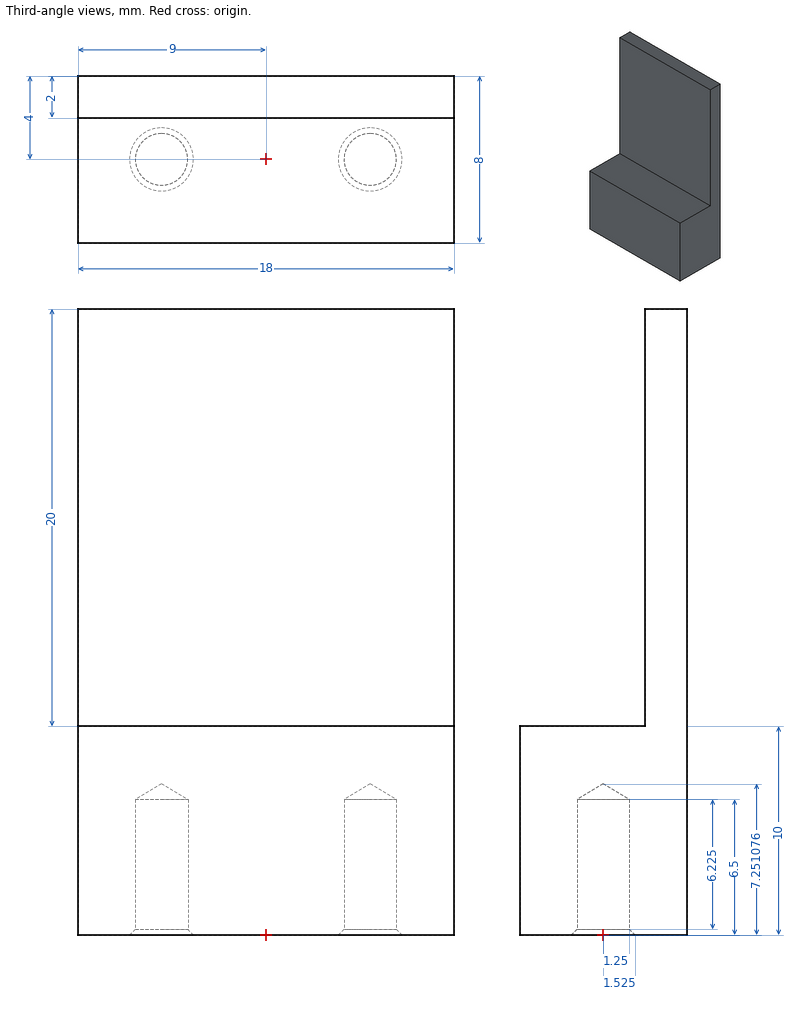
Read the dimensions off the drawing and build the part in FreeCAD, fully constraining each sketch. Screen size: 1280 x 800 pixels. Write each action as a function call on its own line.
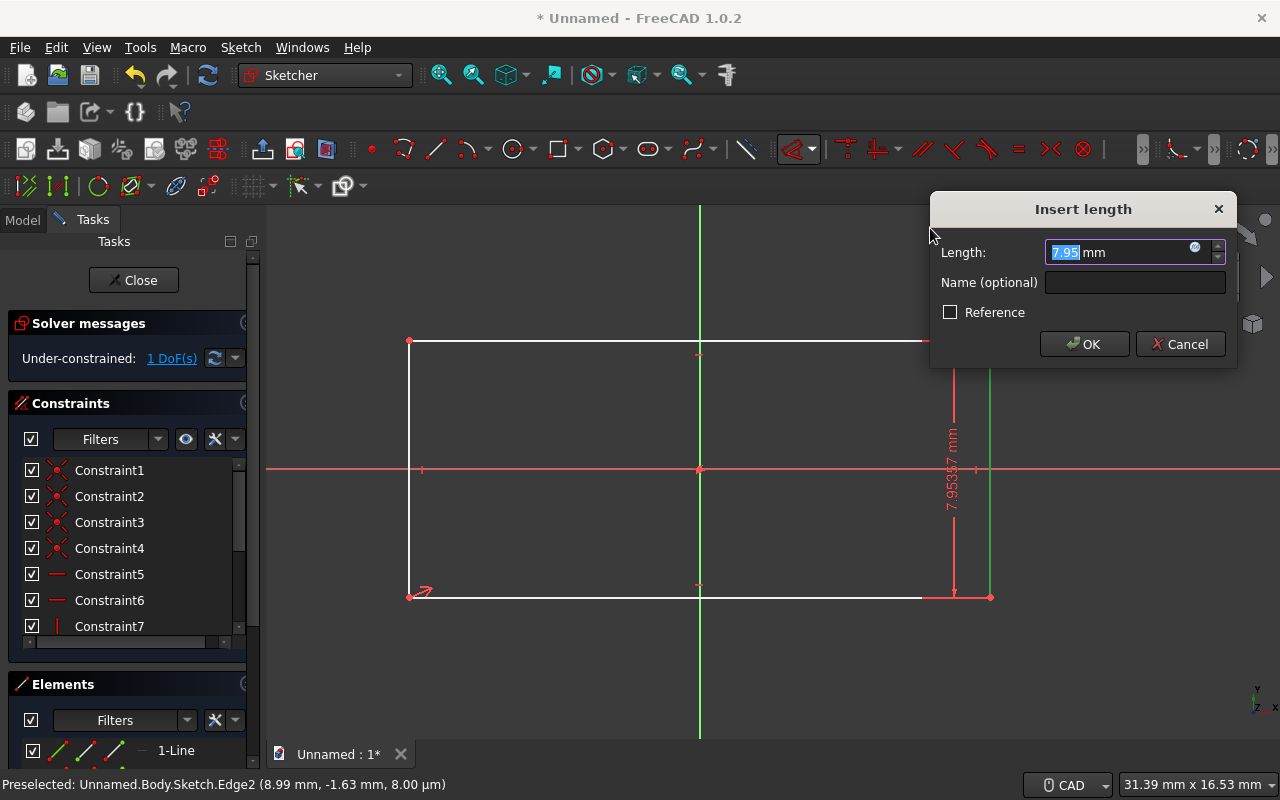
text(8)
key(Return)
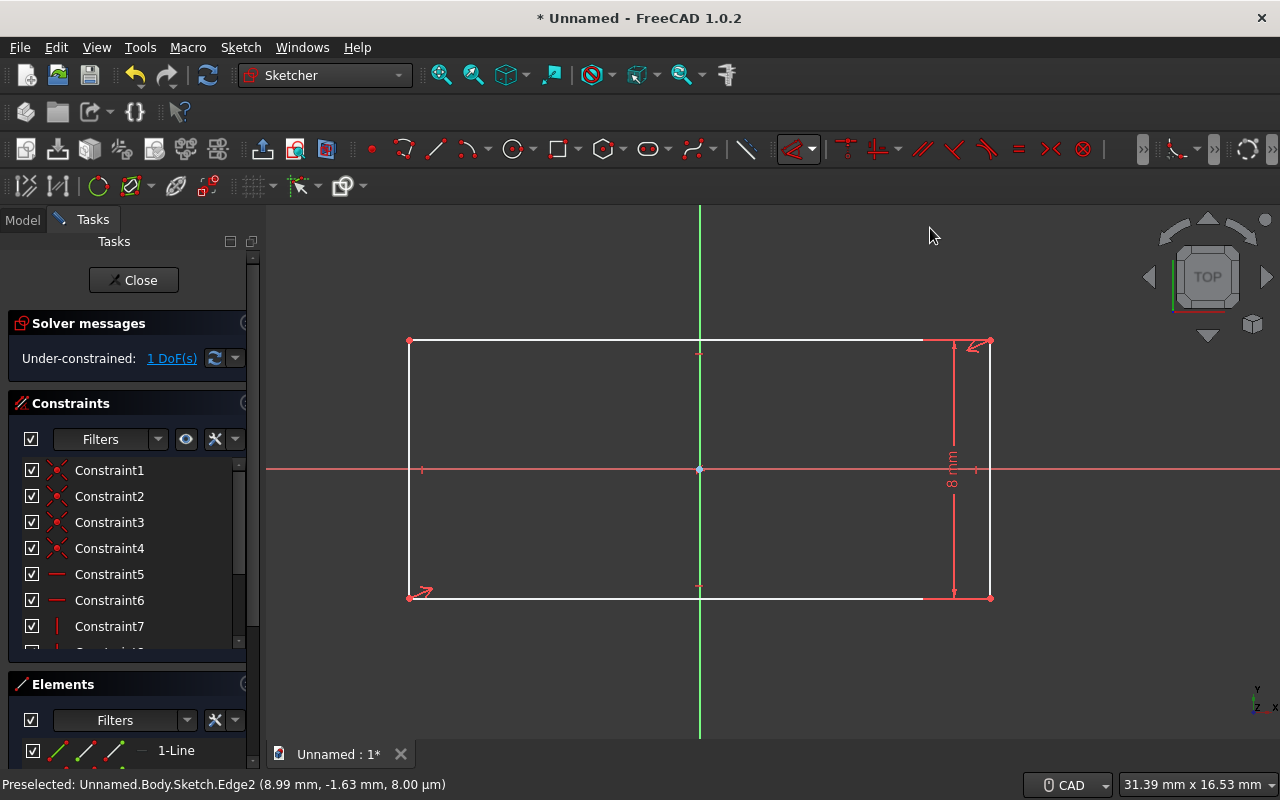
click(584, 599)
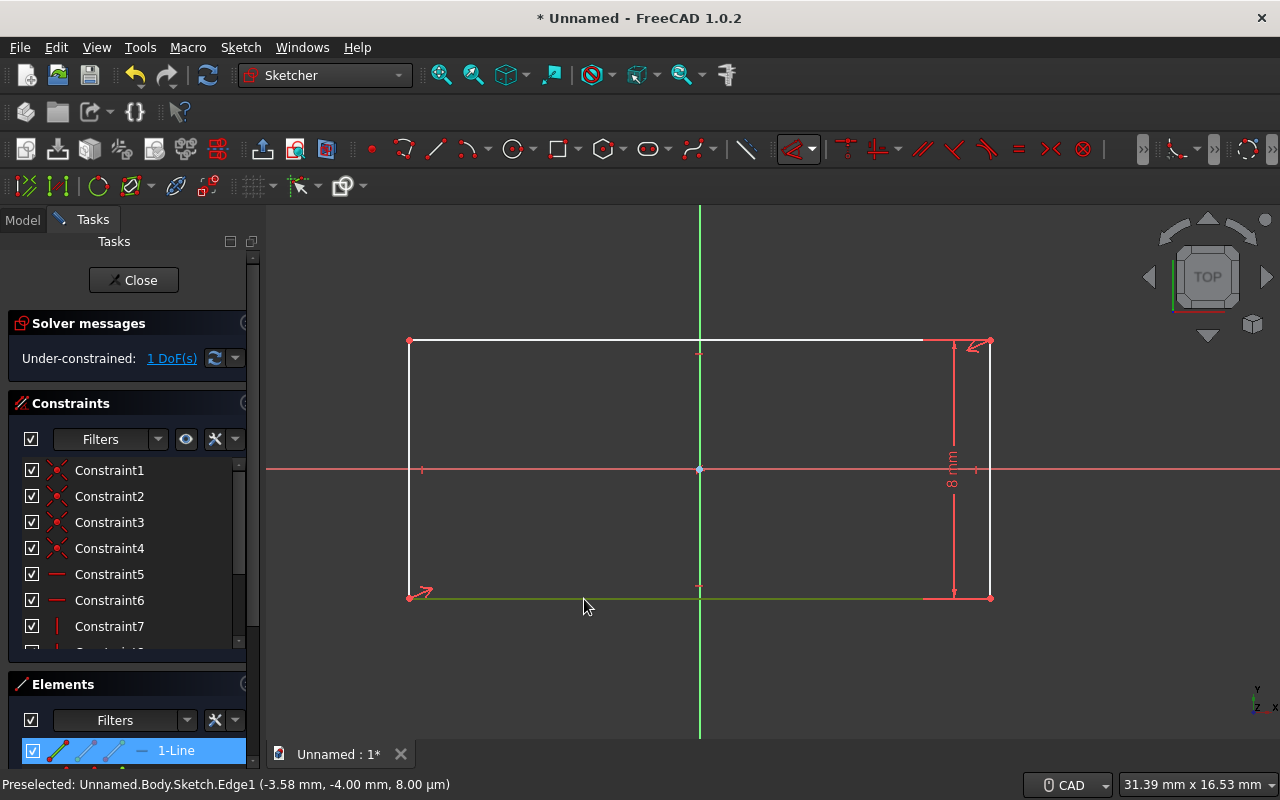
key(l)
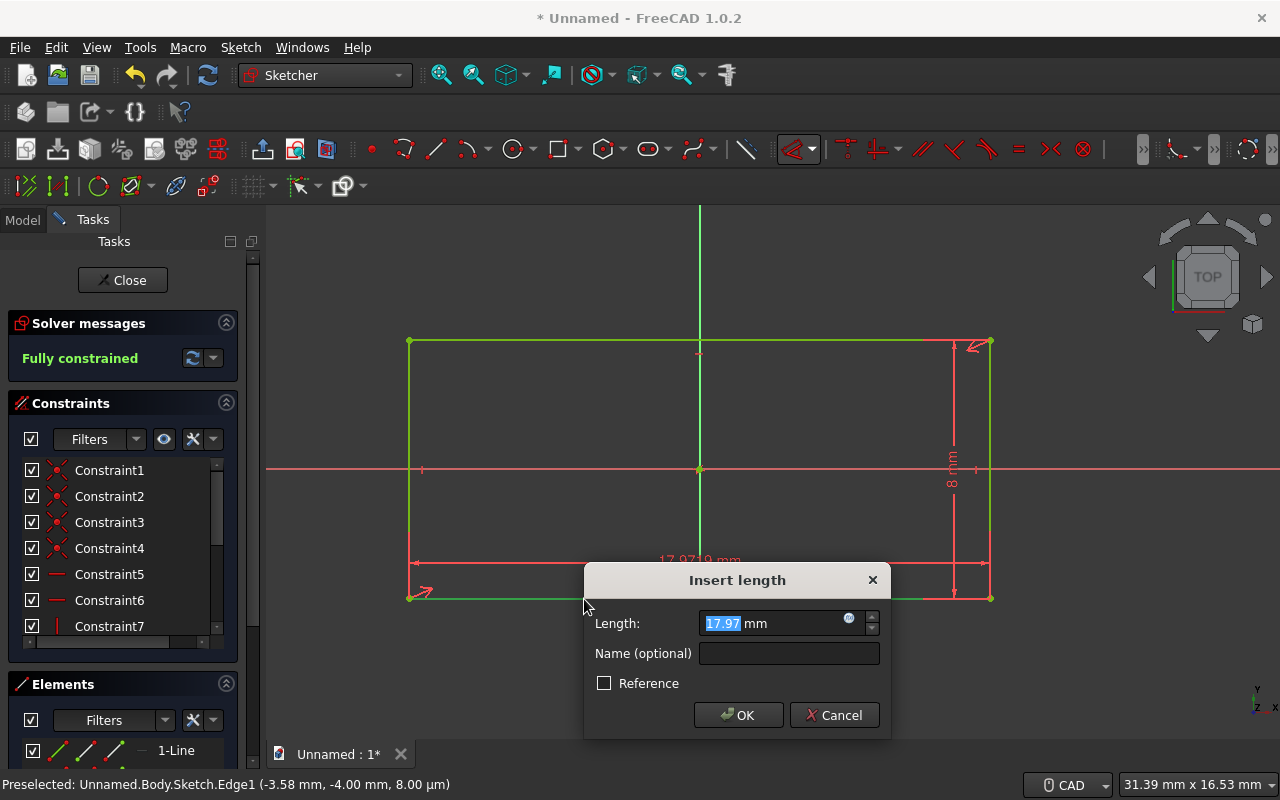
text(18)
key(Return)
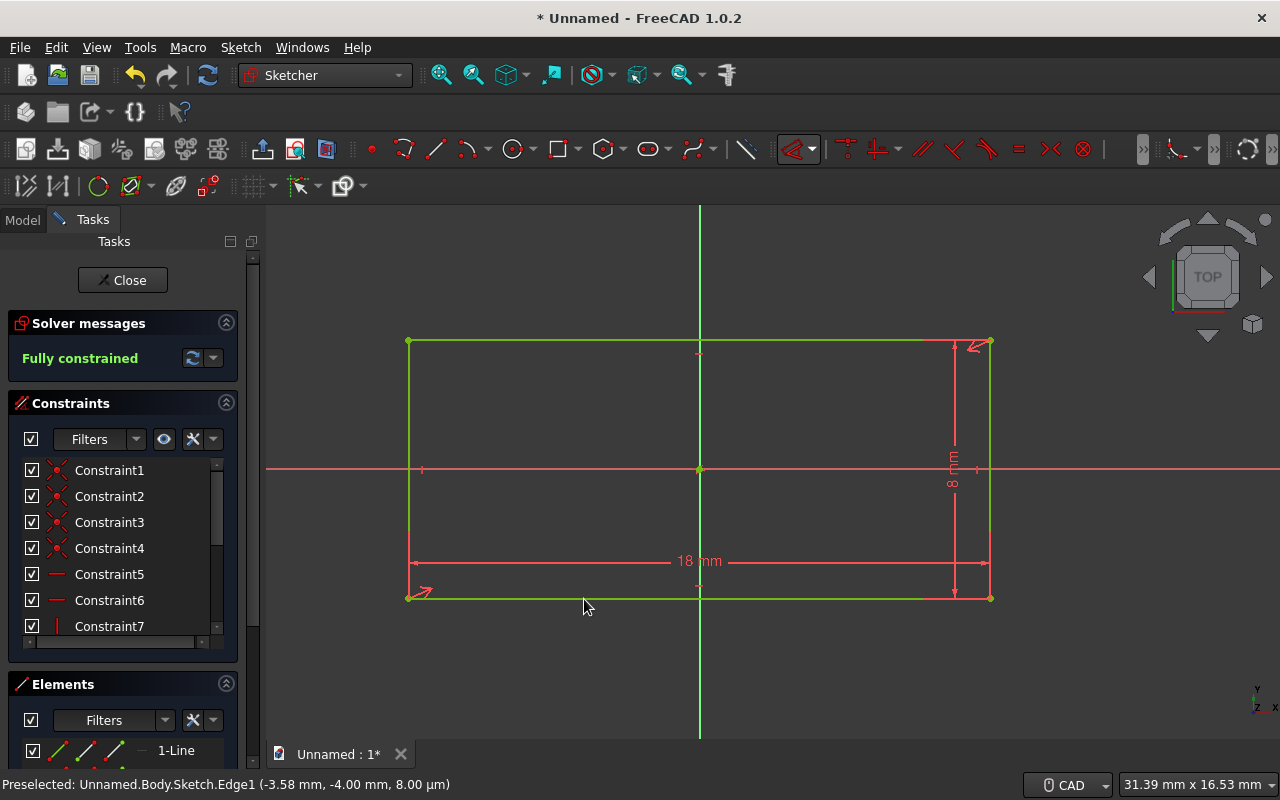
click(123, 280)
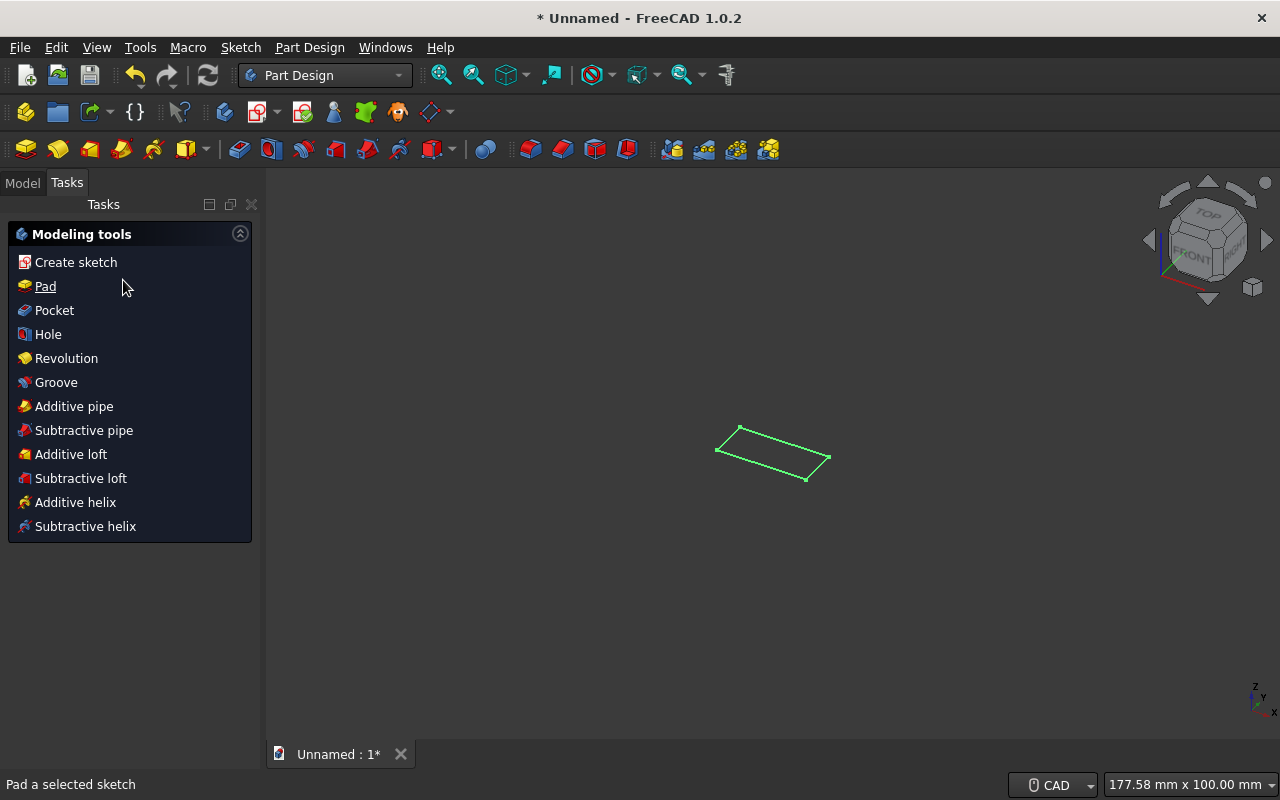
click(26, 150)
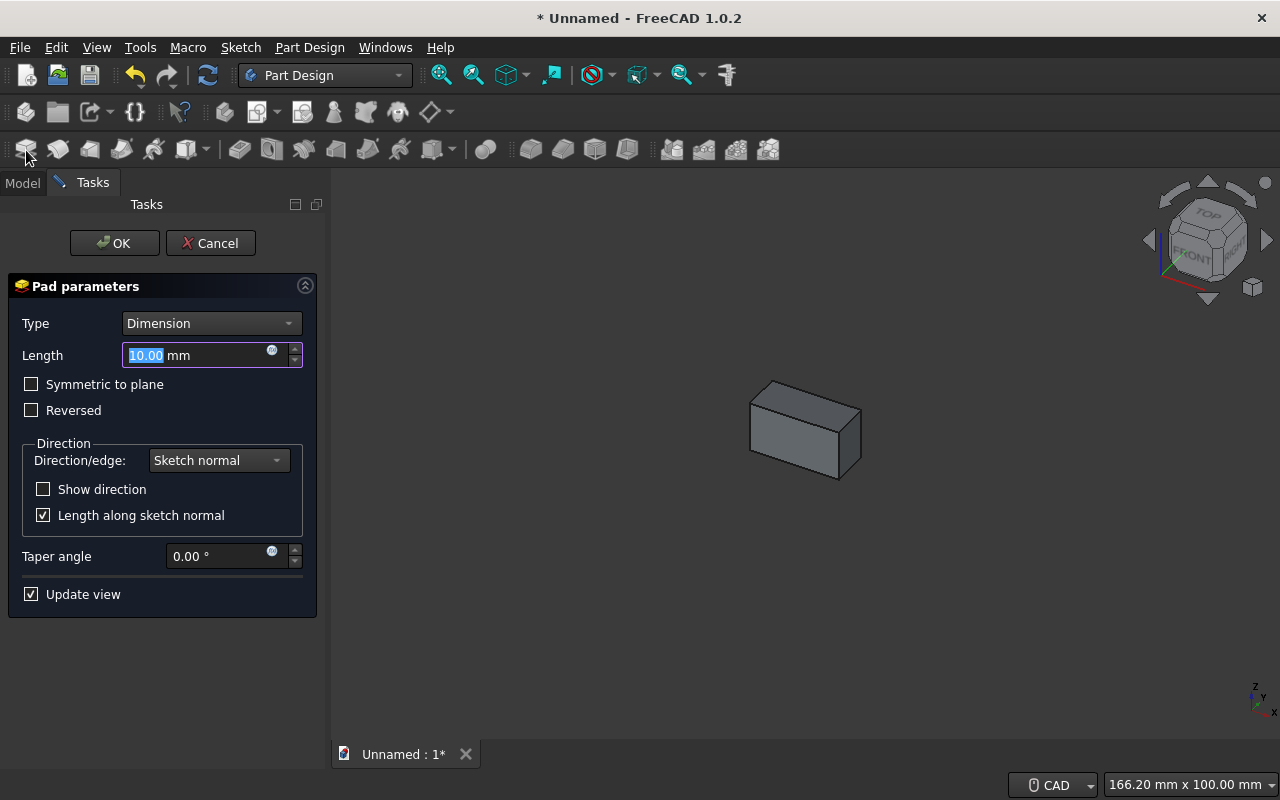
text(10)
key(Tab)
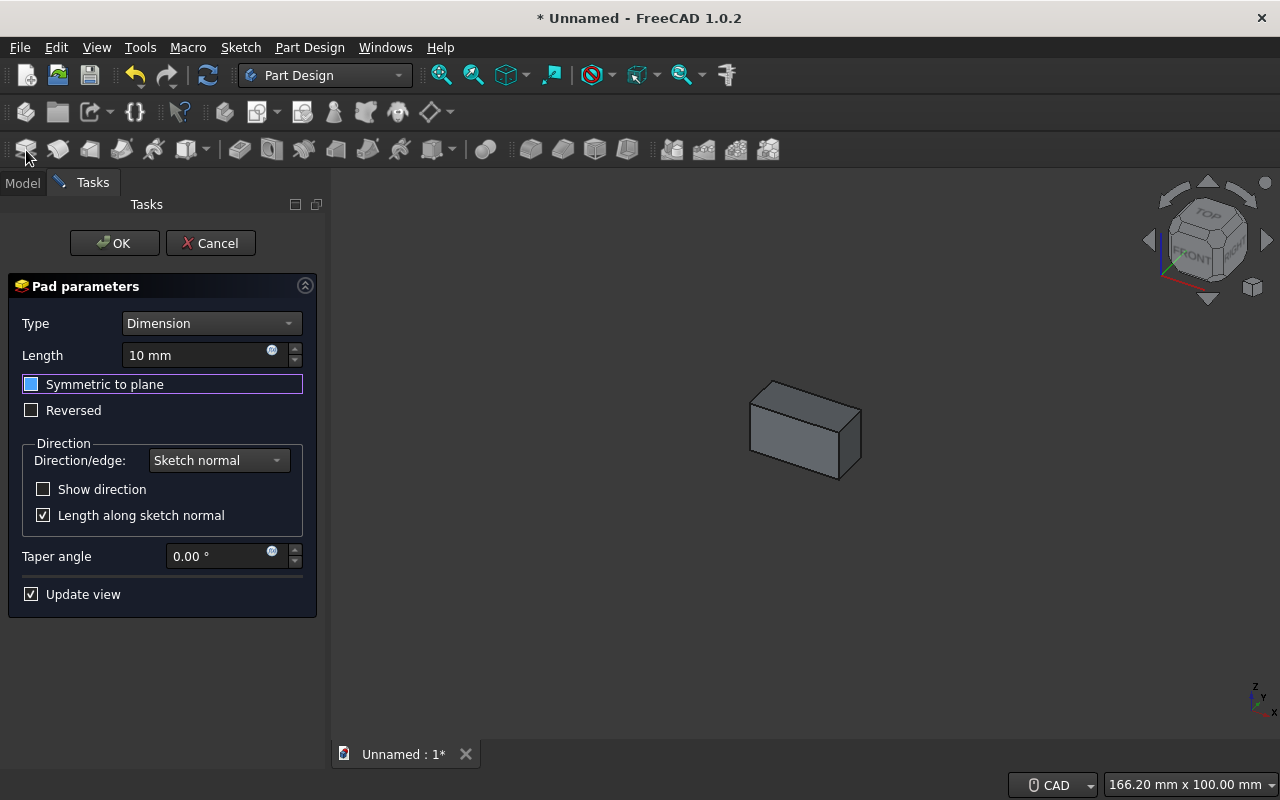
click(115, 243)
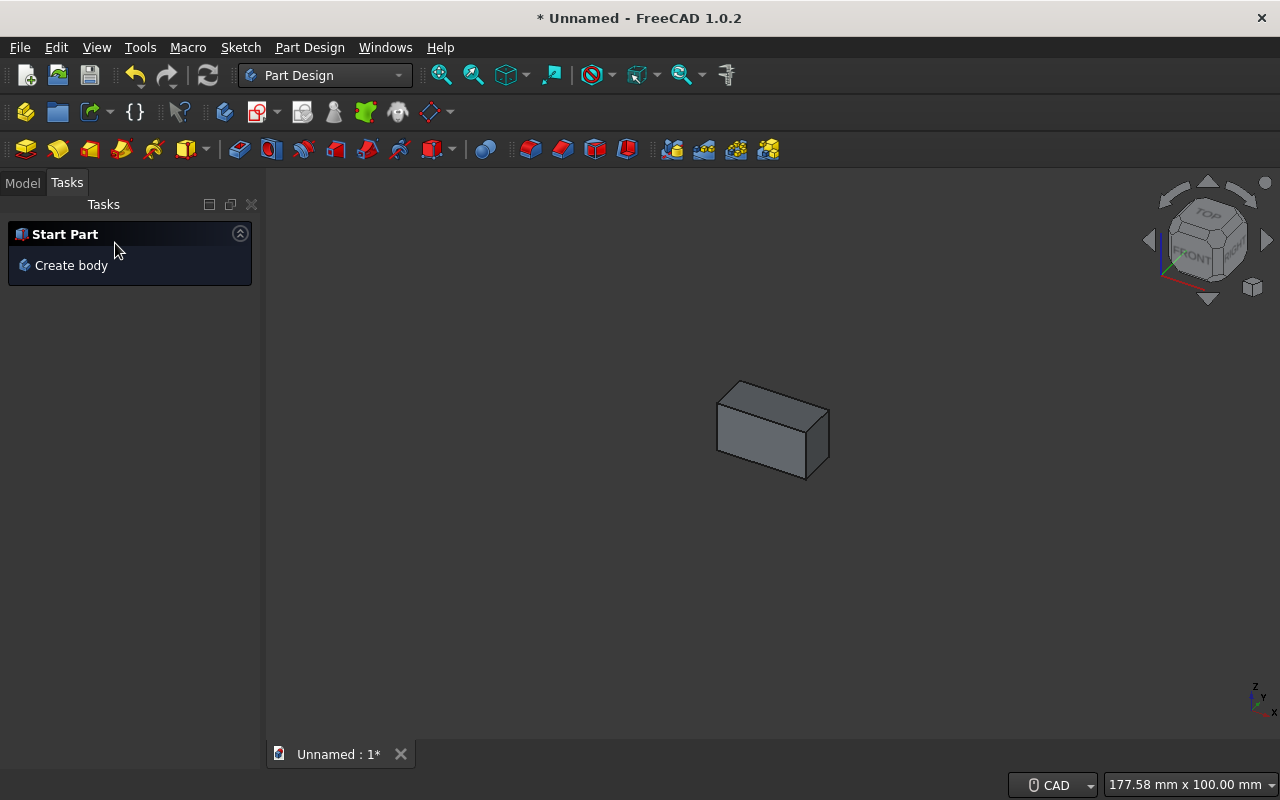
click(442, 76)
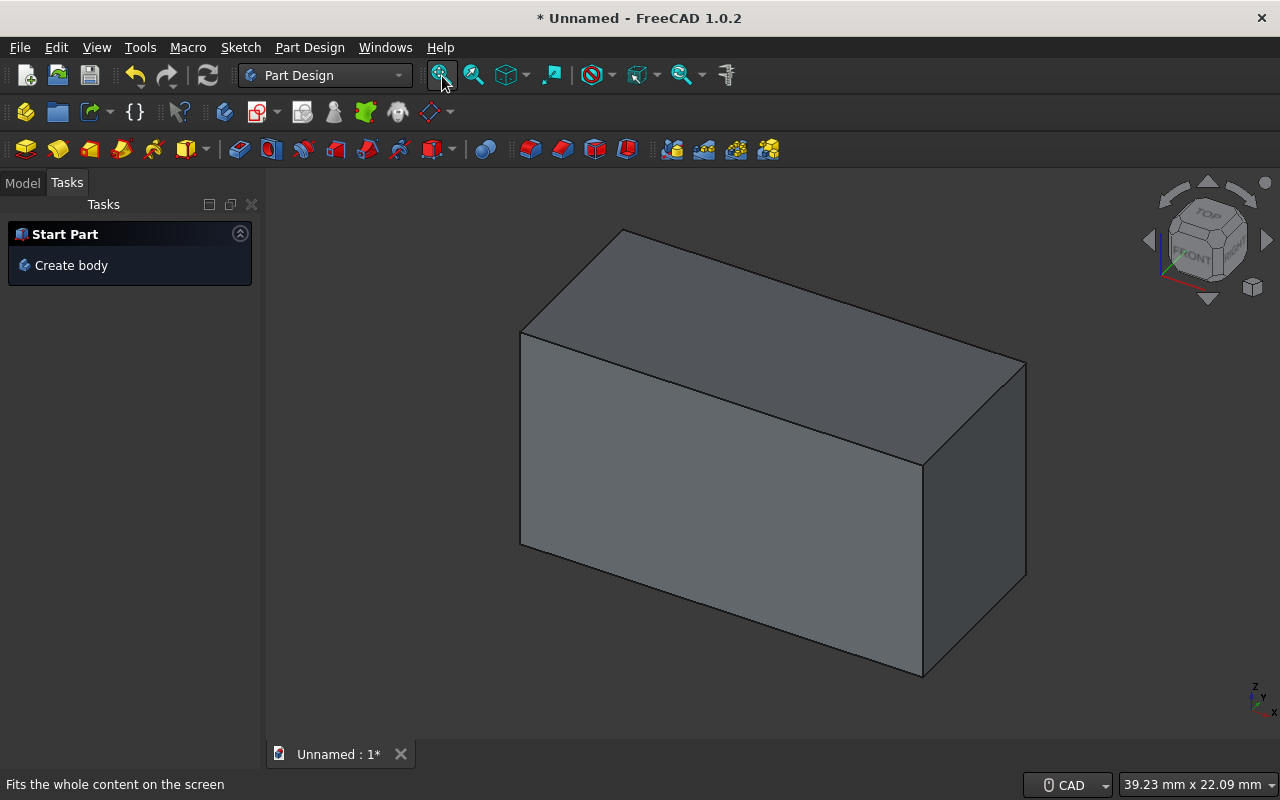
click(831, 366)